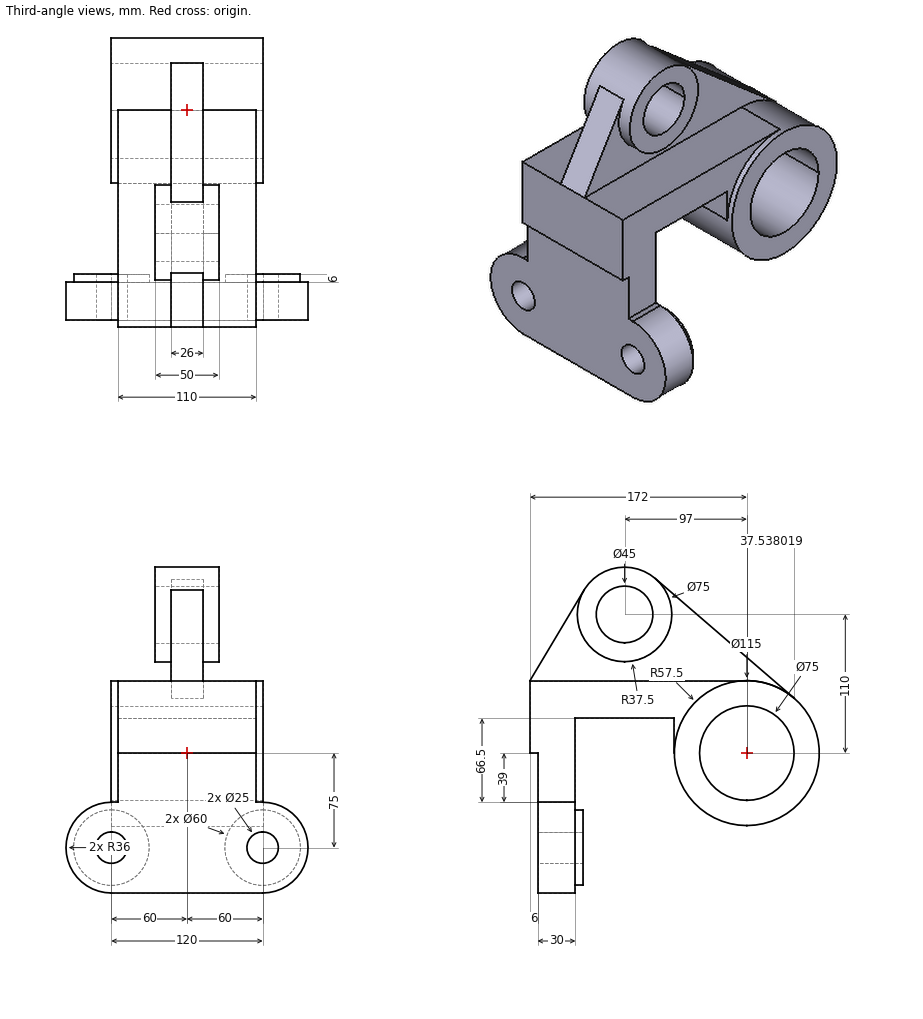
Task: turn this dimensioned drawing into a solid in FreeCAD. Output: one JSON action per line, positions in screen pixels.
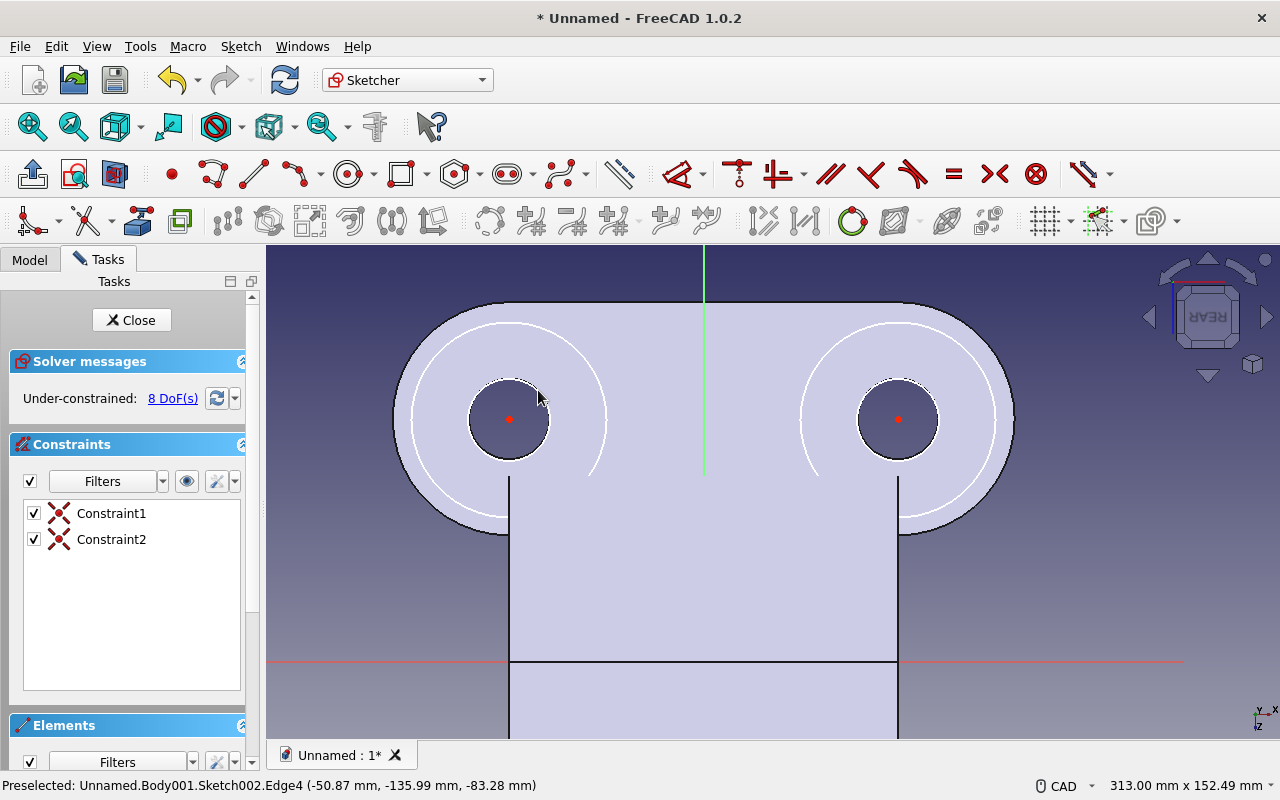
{"action": "left_click", "coordinate": [967, 351]}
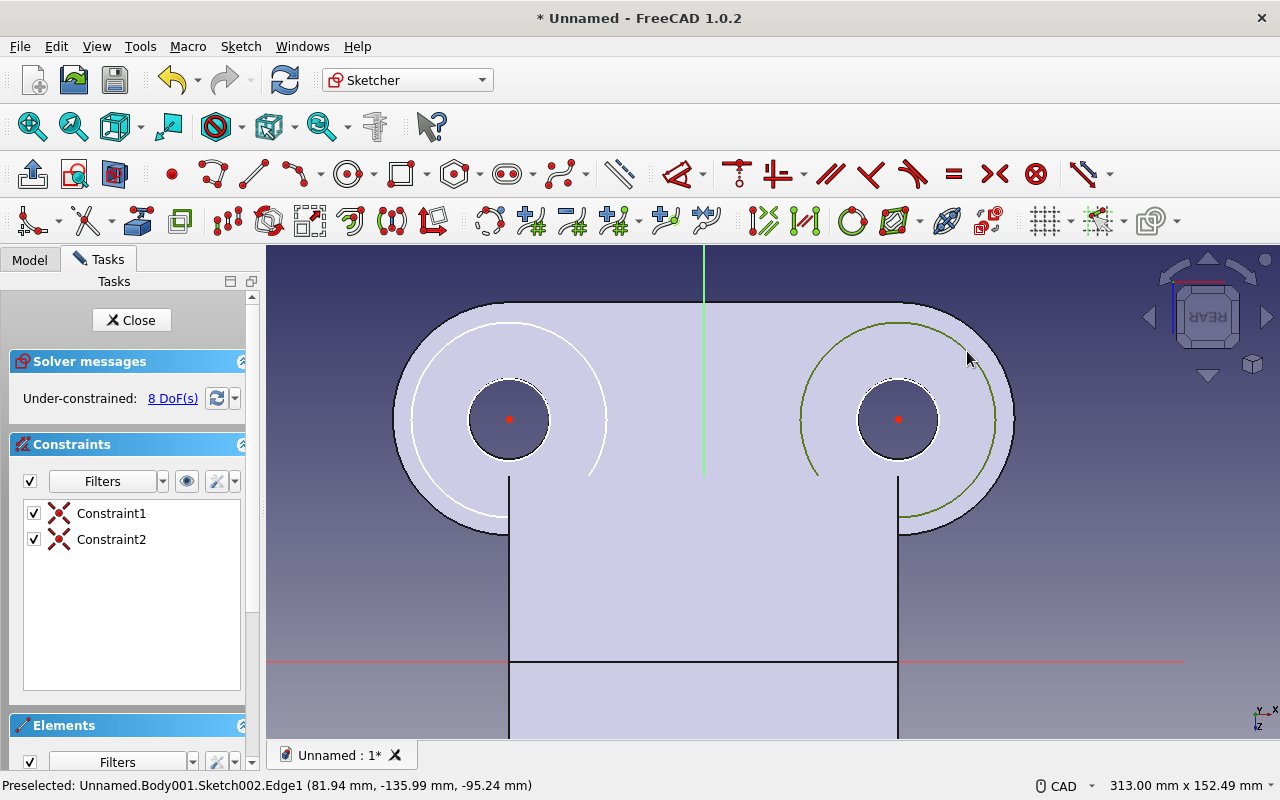
{"action": "left_click", "coordinate": [578, 351]}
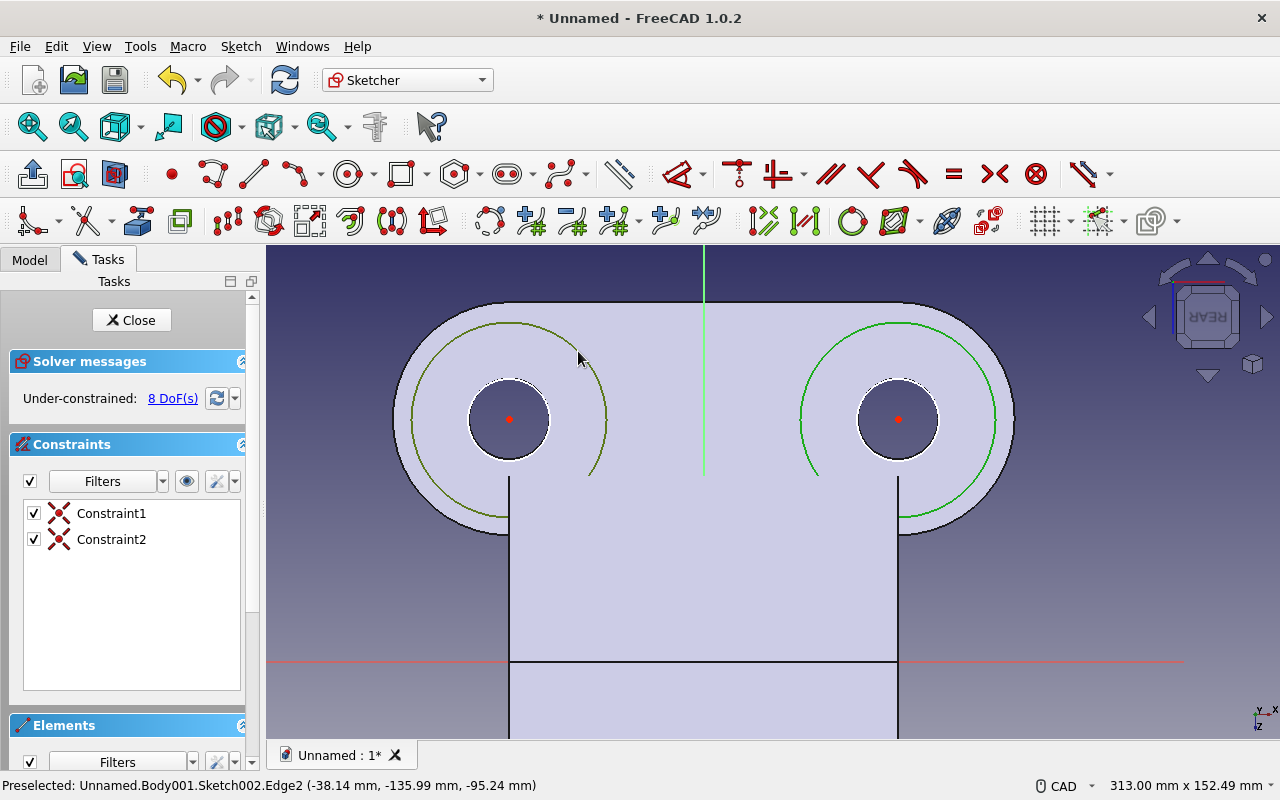
{"action": "key", "text": "e"}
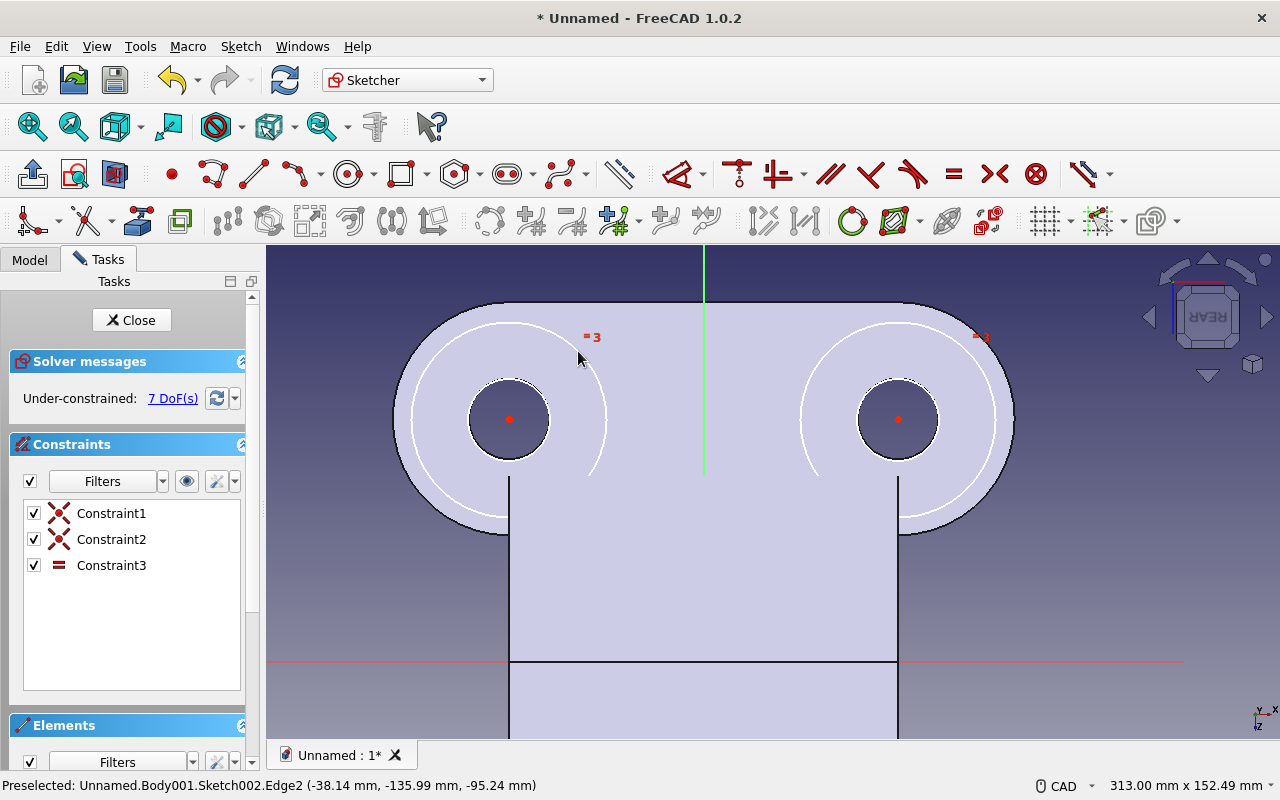
{"action": "left_click", "coordinate": [927, 391]}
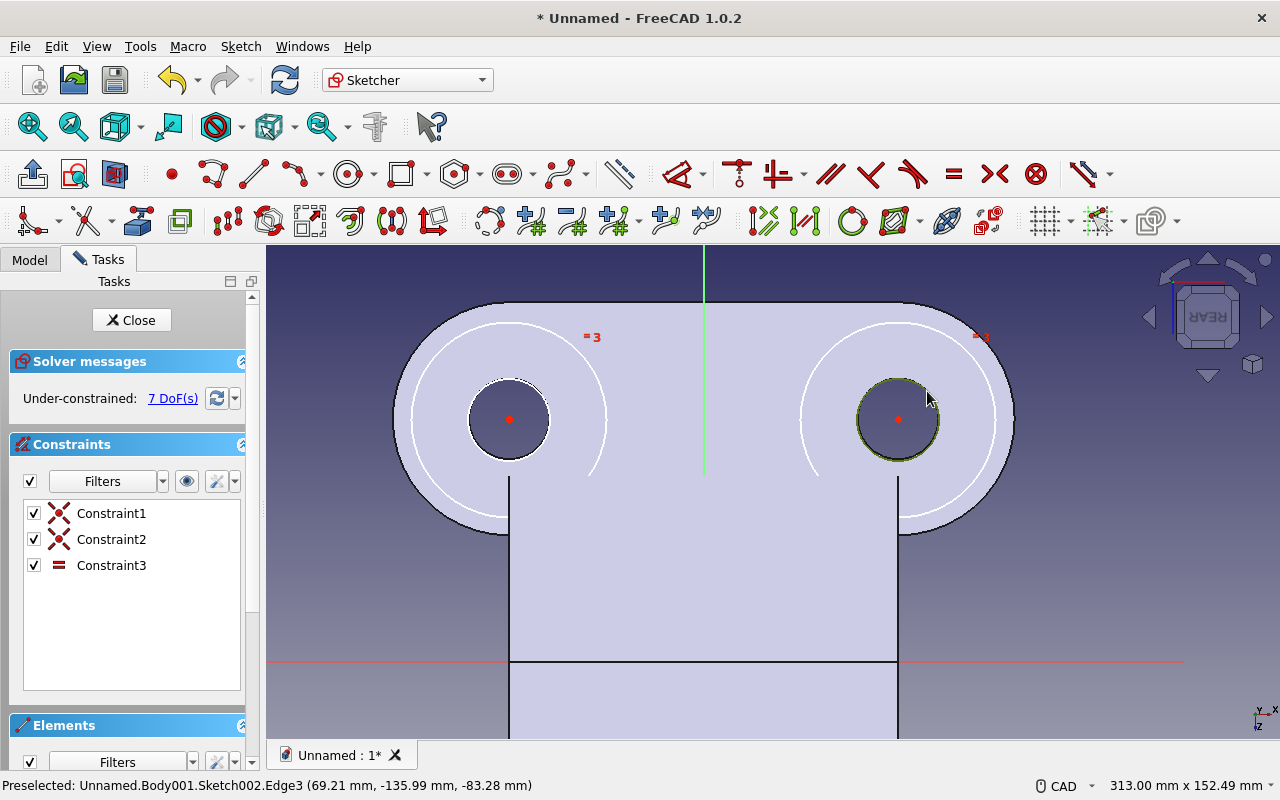
{"action": "left_click", "coordinate": [538, 391]}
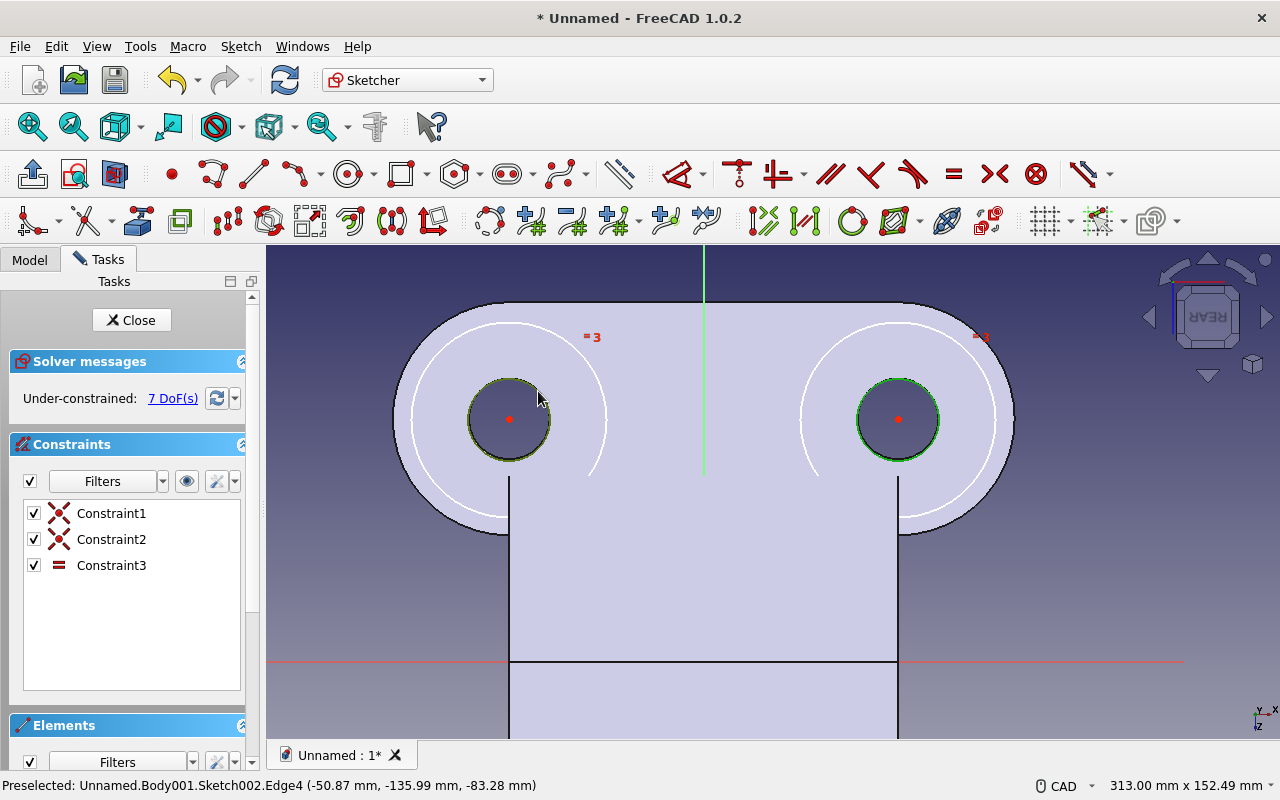
{"action": "left_click", "coordinate": [954, 174]}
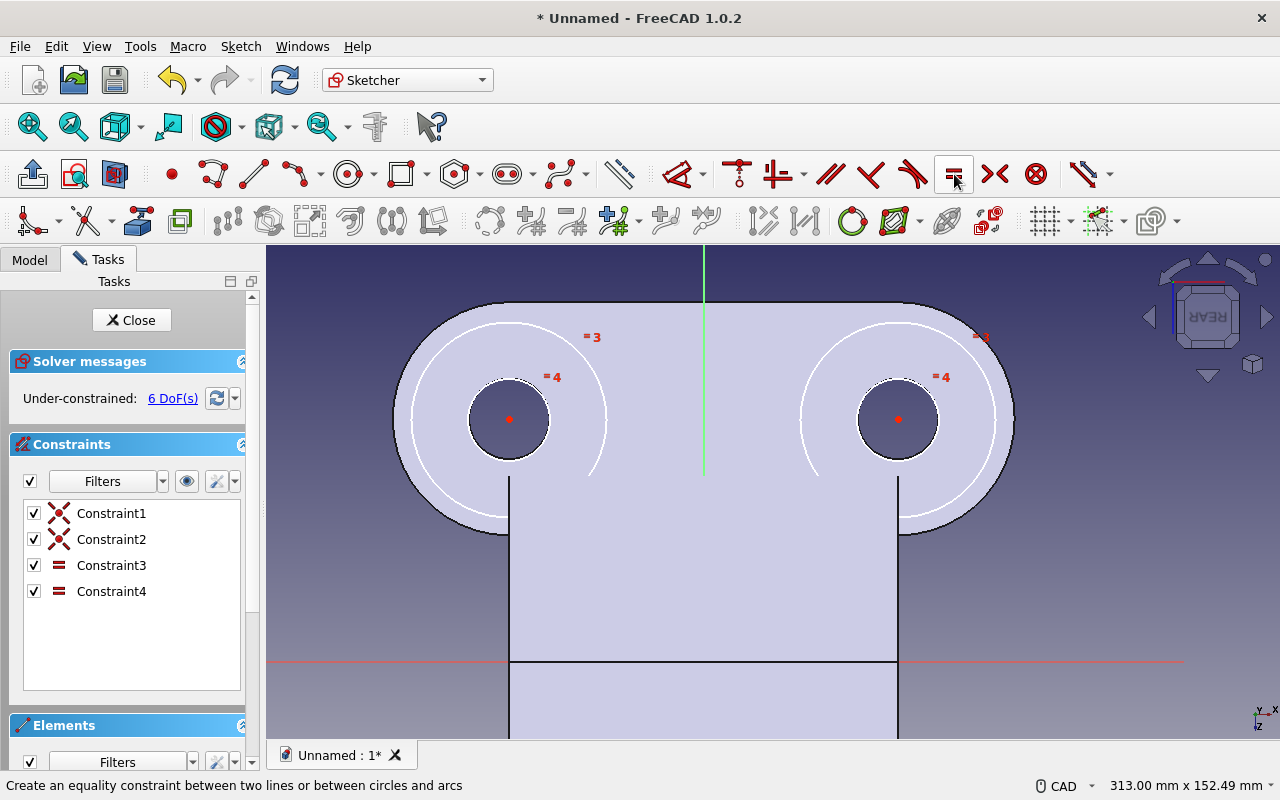
{"action": "left_click", "coordinate": [898, 420]}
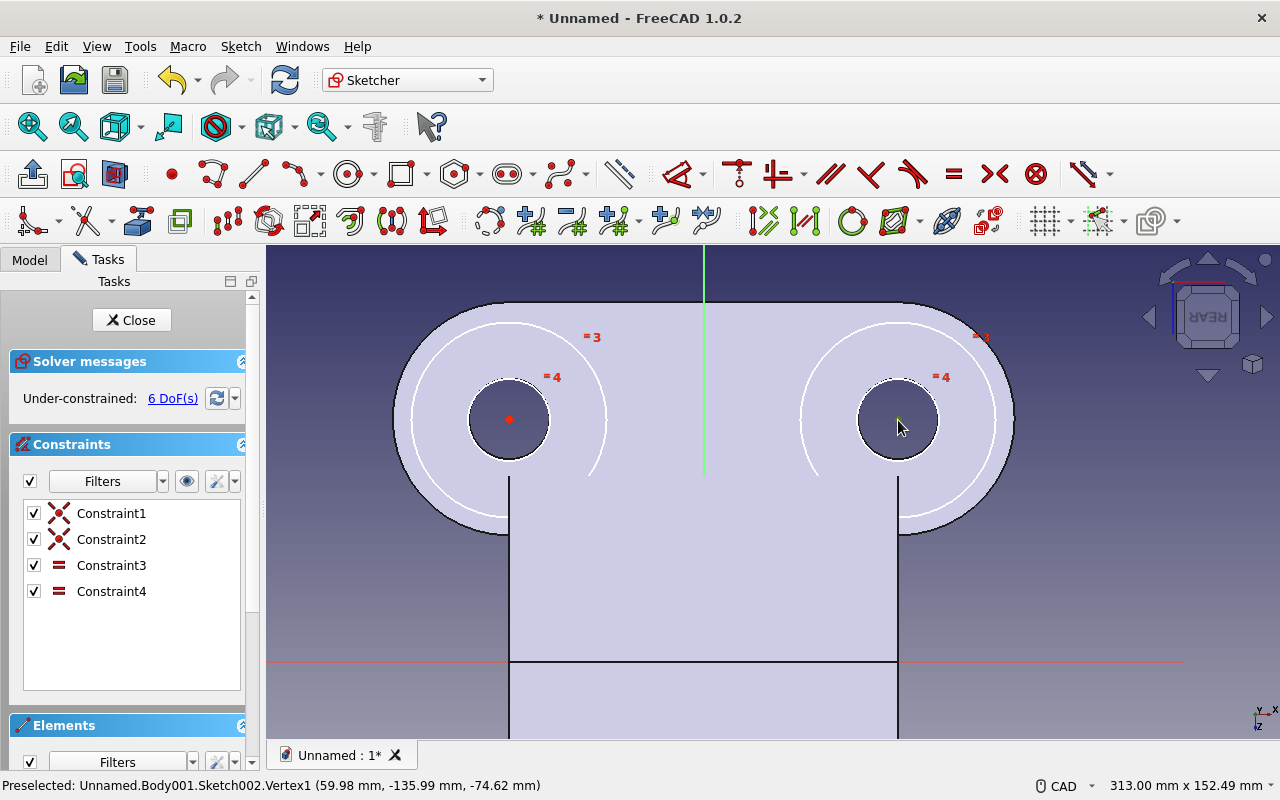
{"action": "left_click", "coordinate": [509, 420]}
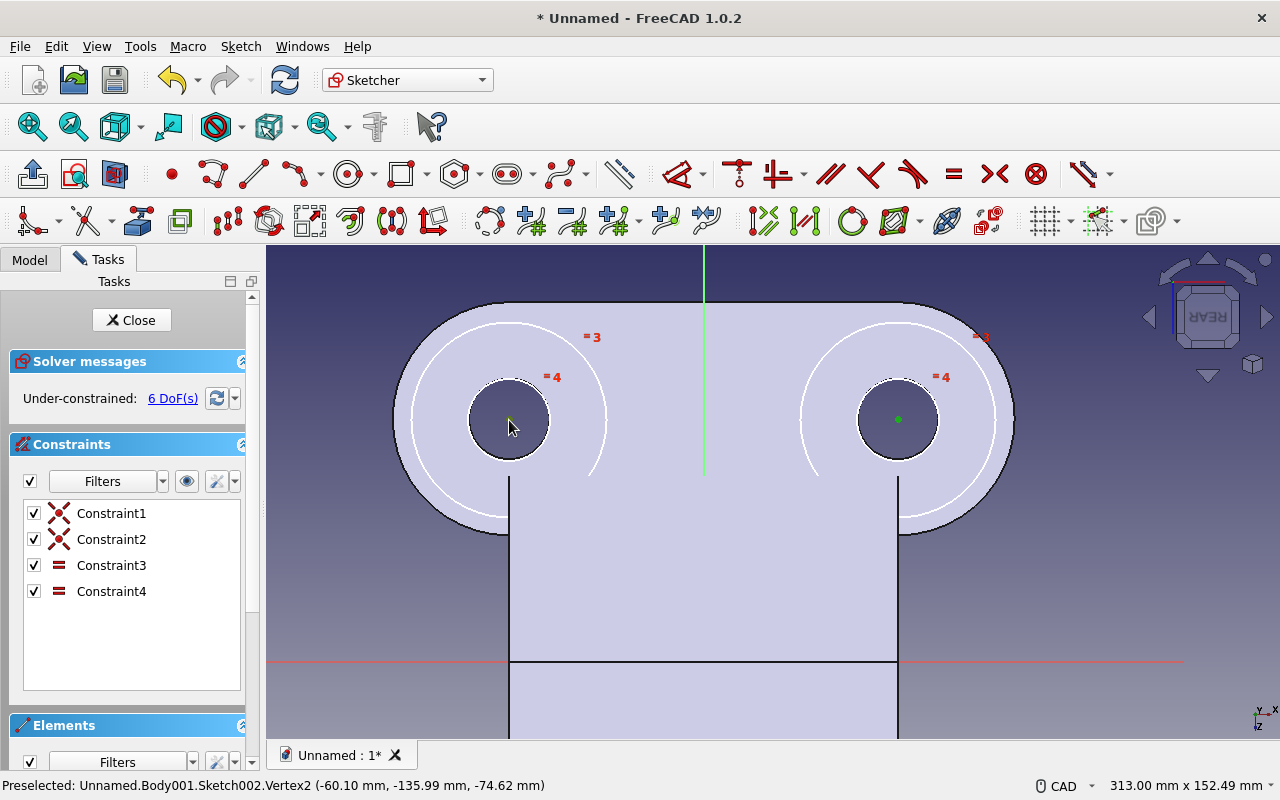
{"action": "left_click", "coordinate": [804, 174]}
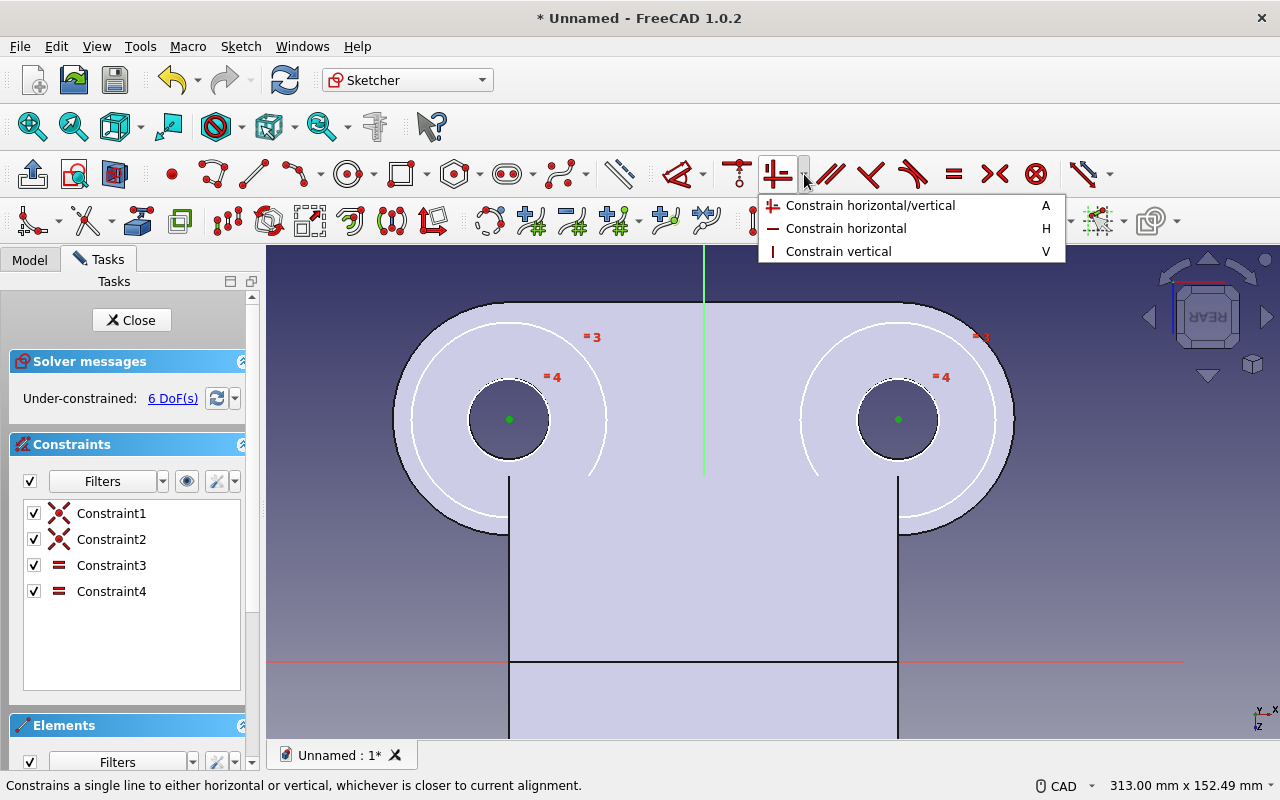
{"action": "left_click", "coordinate": [912, 228]}